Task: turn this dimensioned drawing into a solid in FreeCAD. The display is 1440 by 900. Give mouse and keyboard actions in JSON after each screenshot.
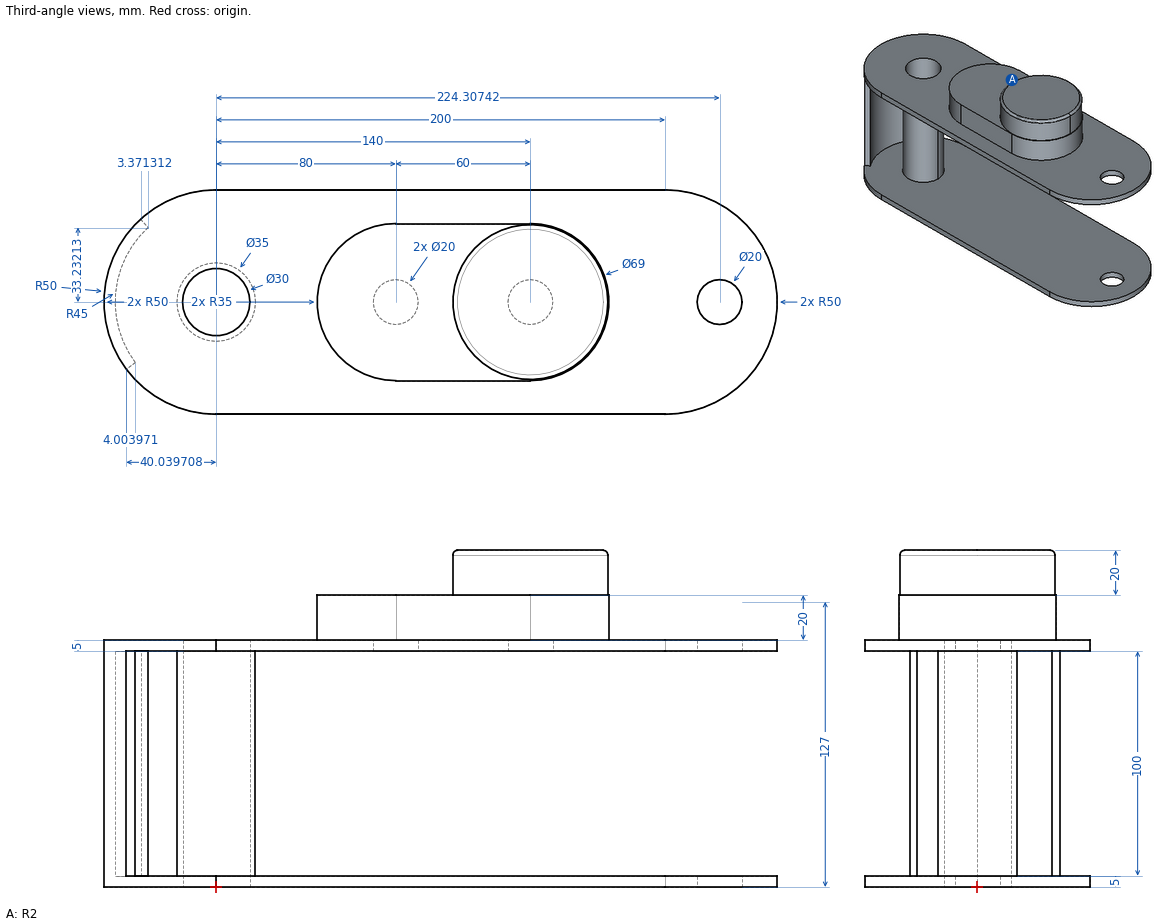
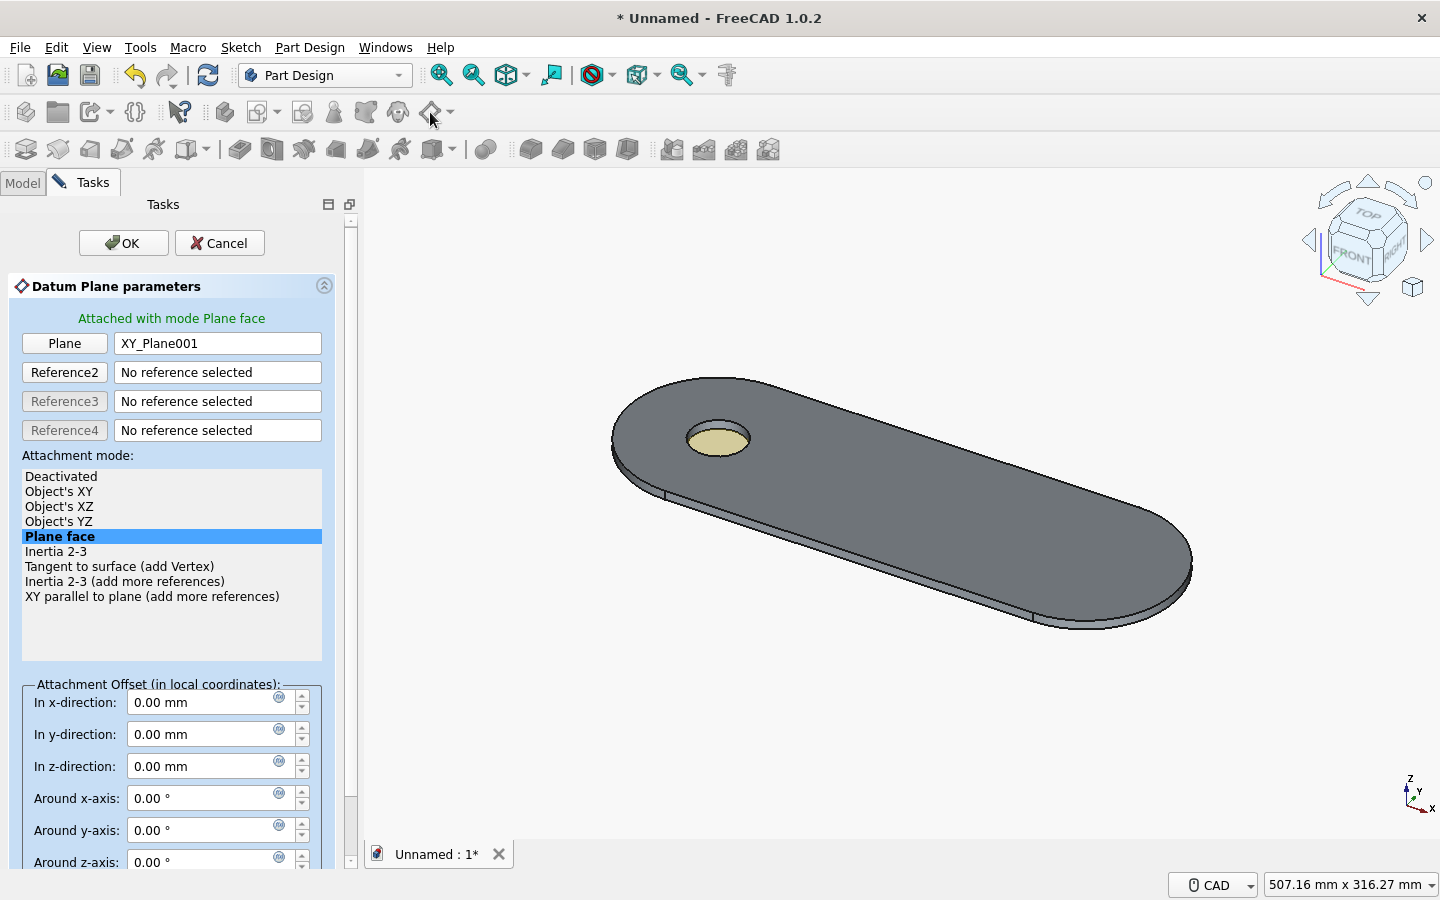
{"action": "triple_click", "coordinate": [210, 766]}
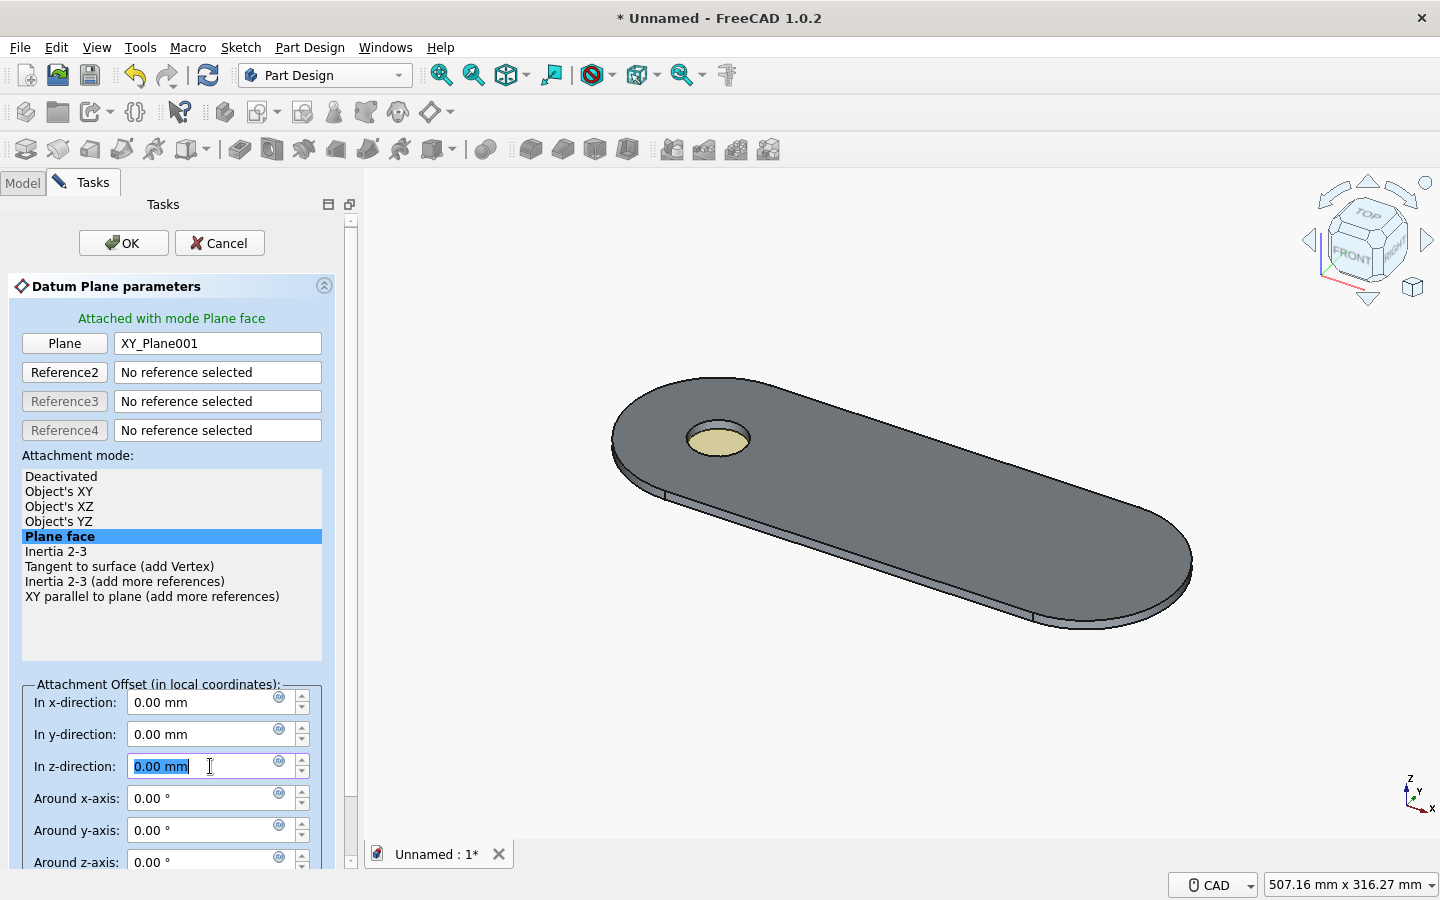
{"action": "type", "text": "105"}
{"action": "key", "text": "Tab"}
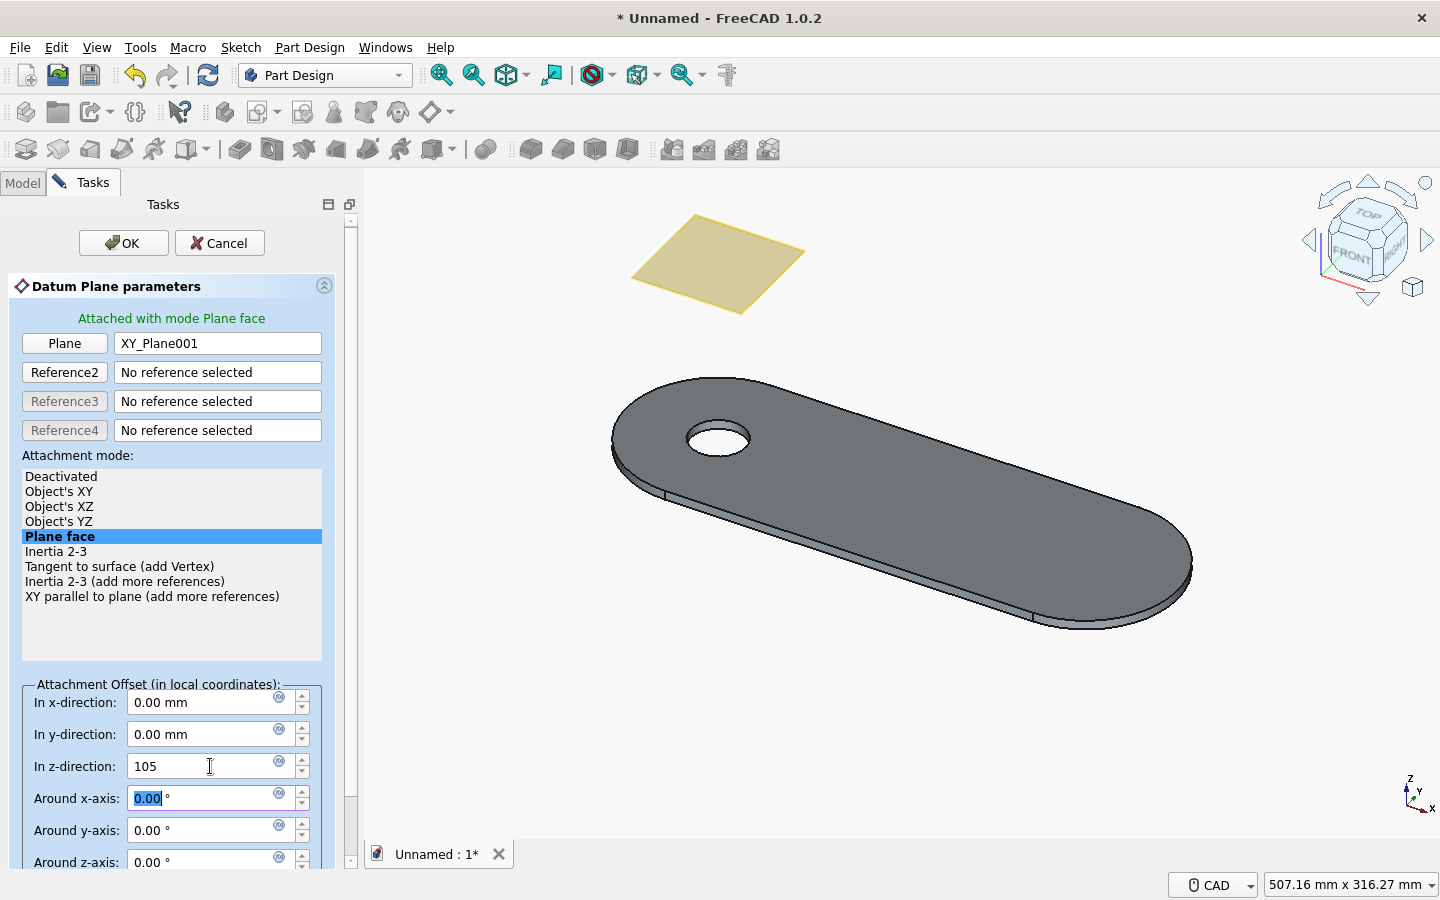
{"action": "left_click", "coordinate": [124, 243]}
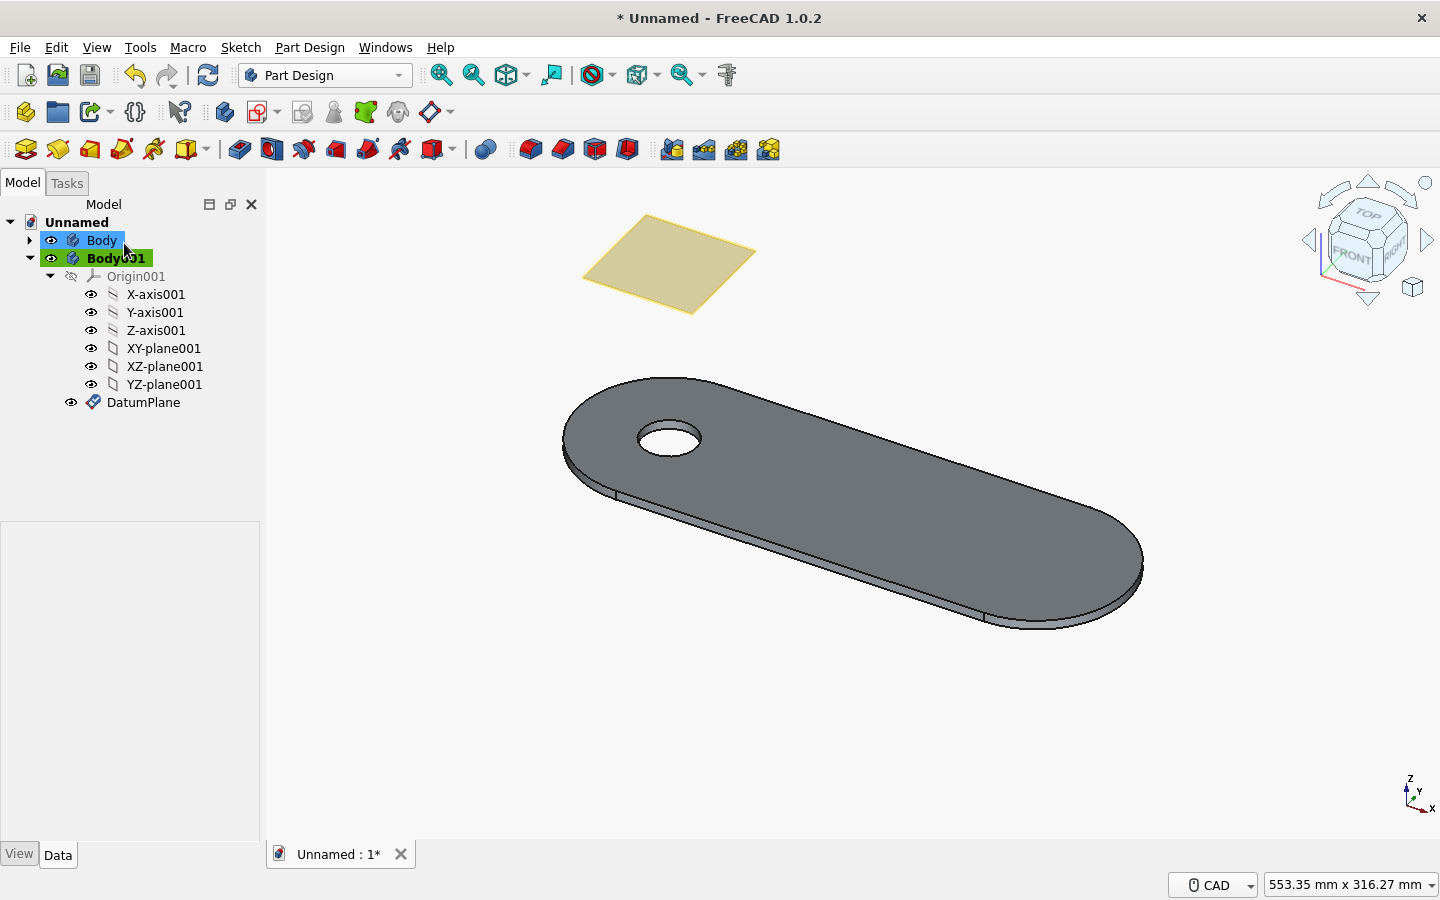
{"action": "left_click", "coordinate": [116, 402]}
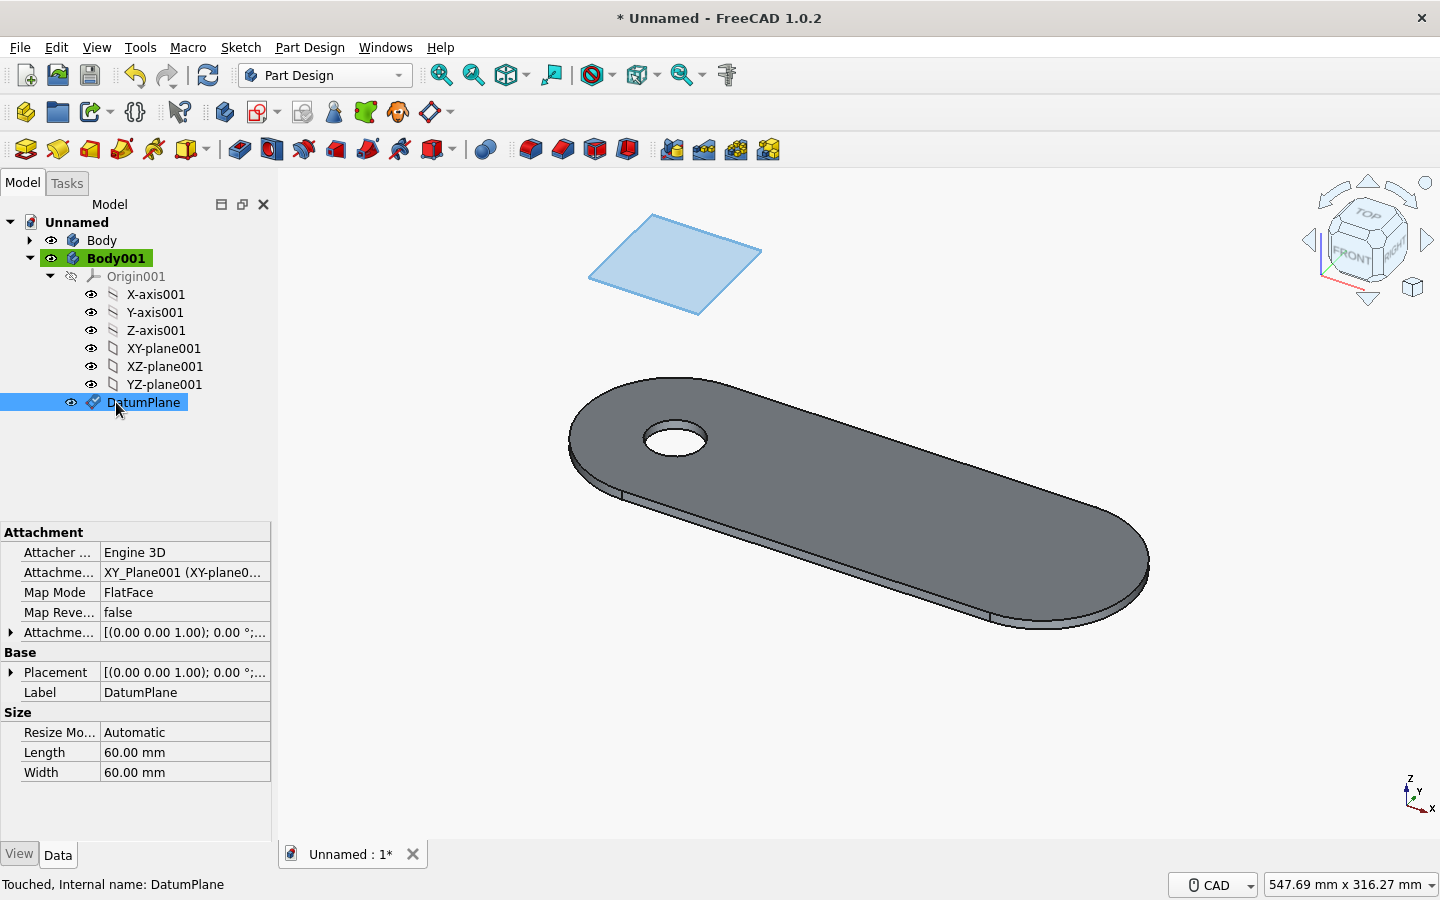
{"action": "left_click", "coordinate": [258, 112]}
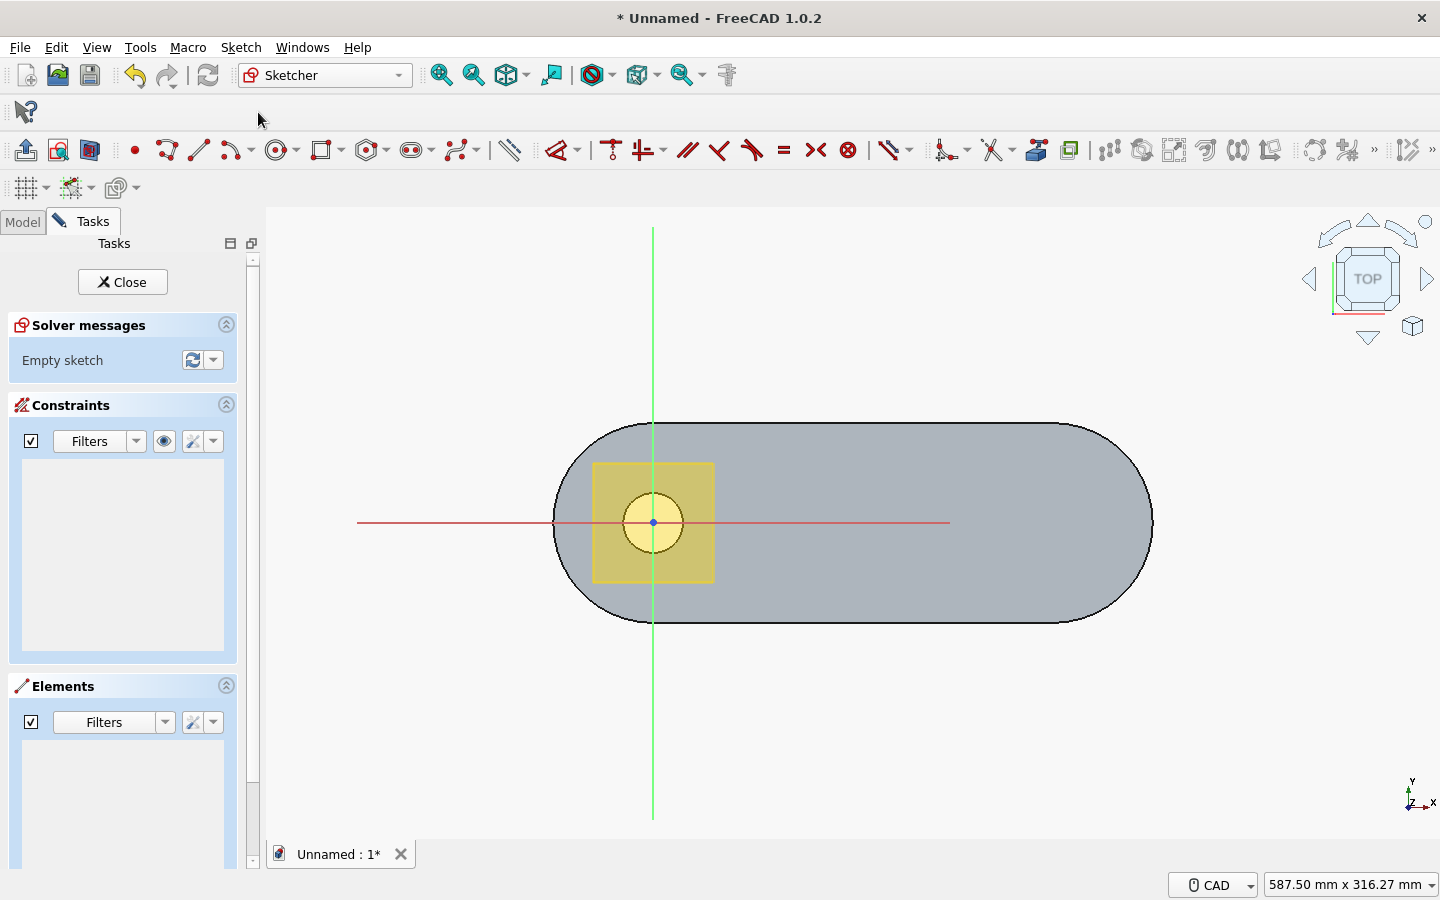
{"action": "left_click", "coordinate": [412, 150]}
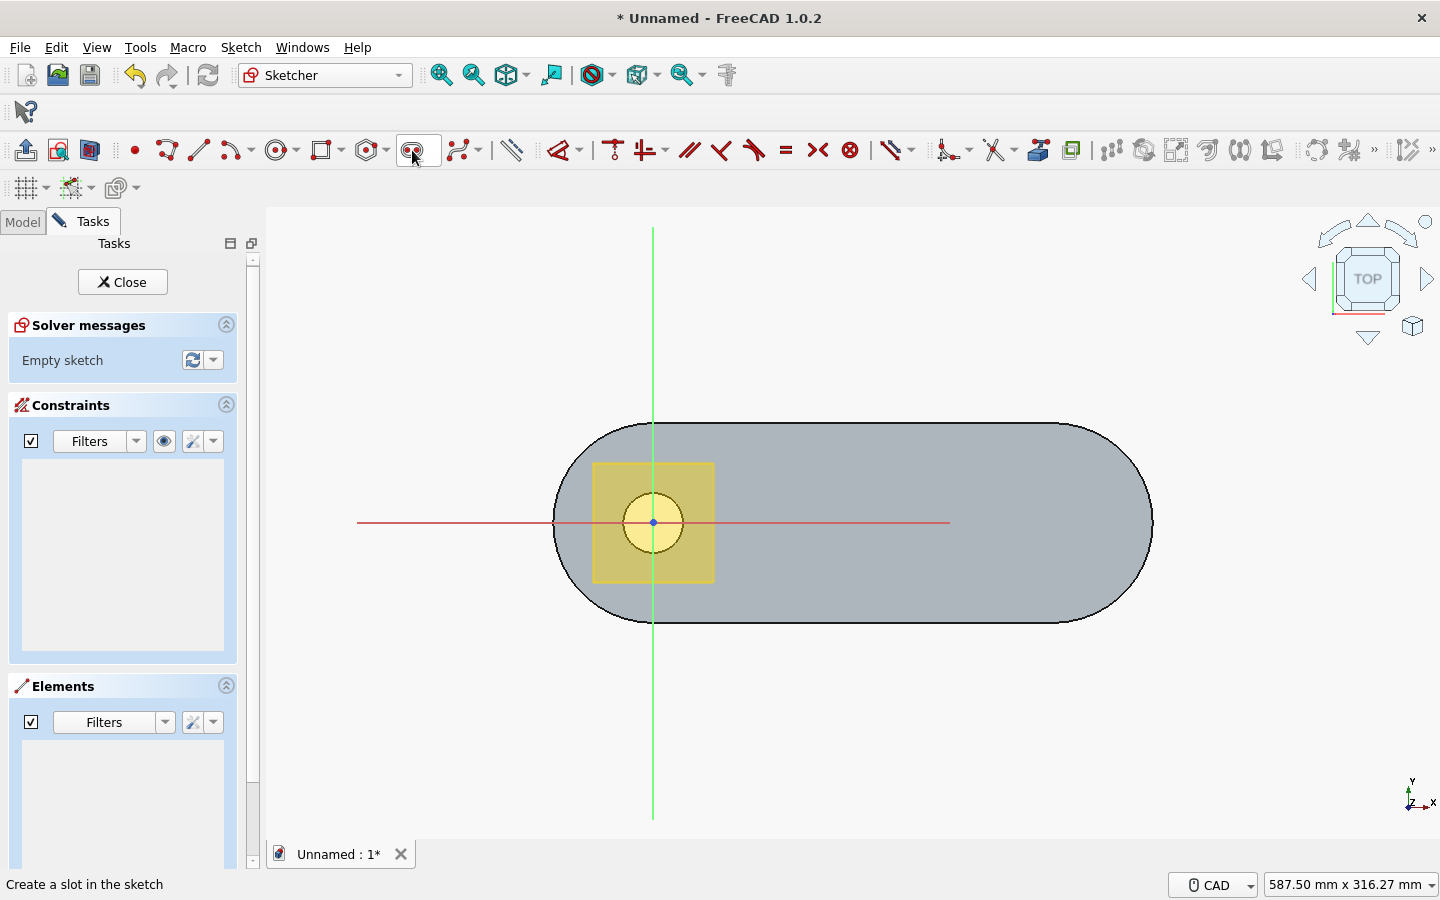
{"action": "left_click", "coordinate": [653, 523]}